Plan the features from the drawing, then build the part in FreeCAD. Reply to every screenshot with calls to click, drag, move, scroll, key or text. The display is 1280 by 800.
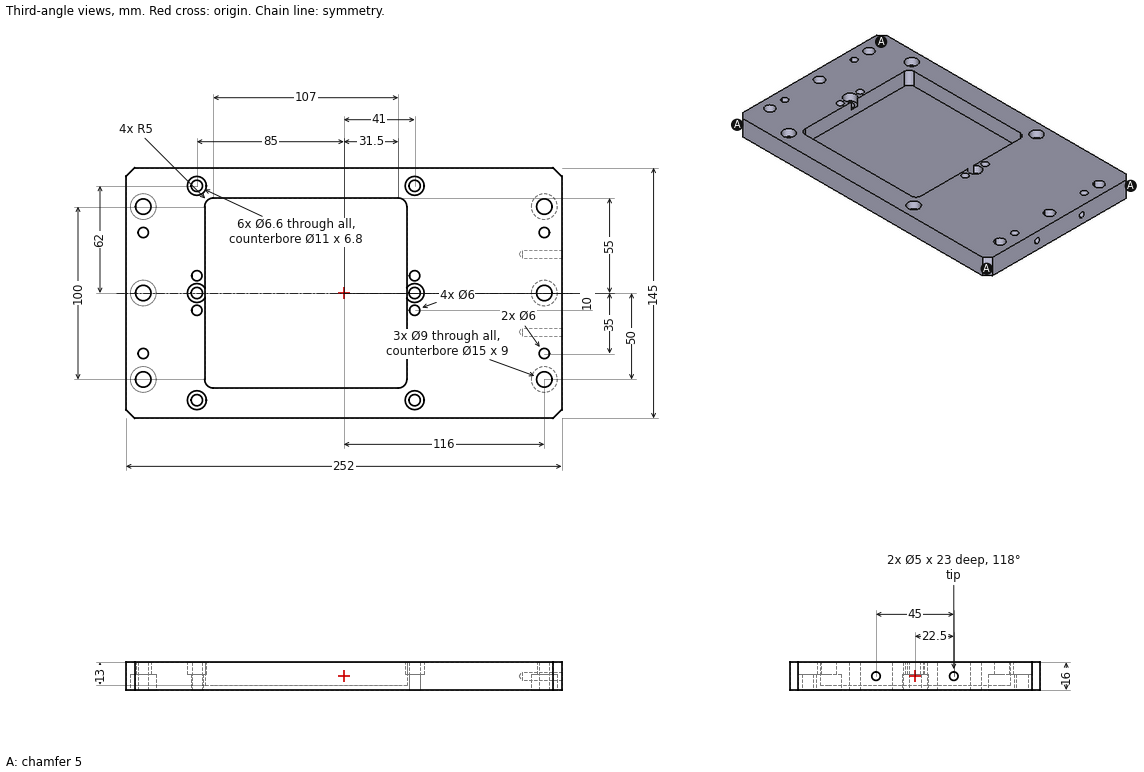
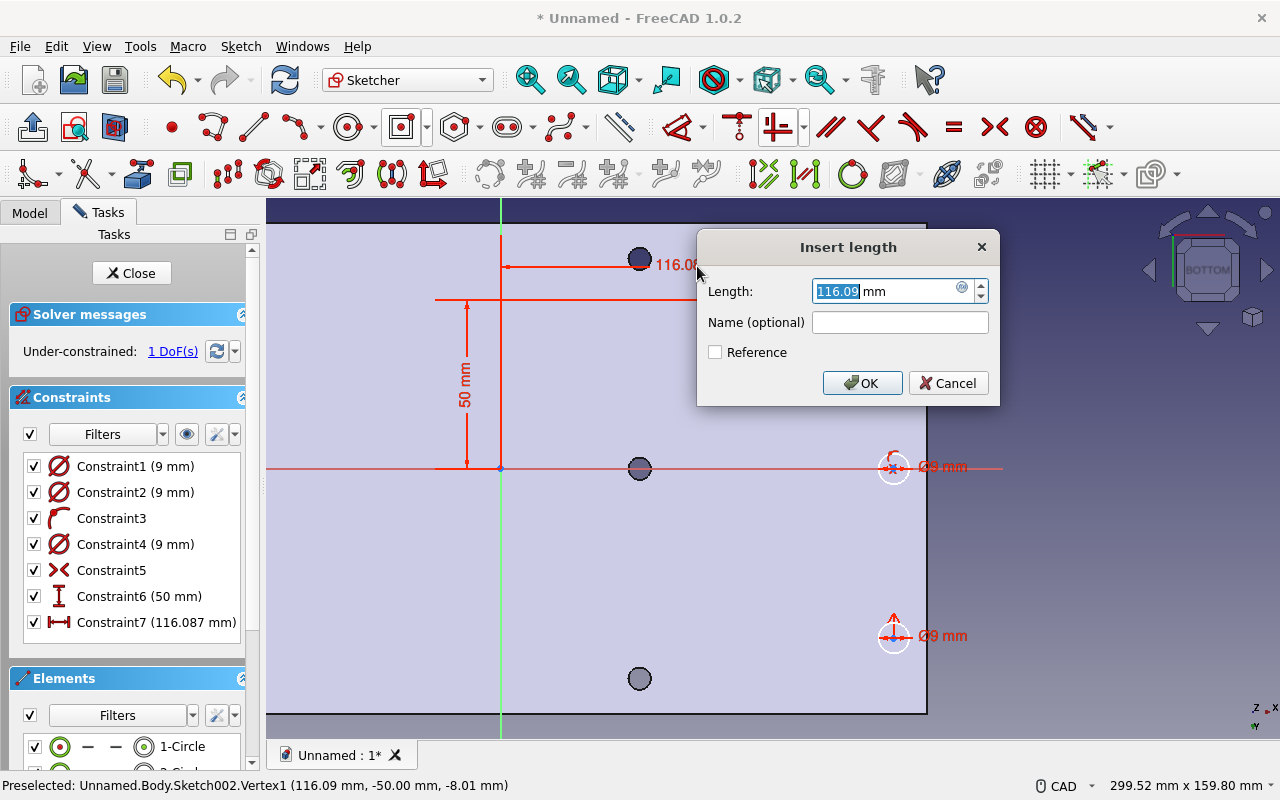
text(116)
key(Return)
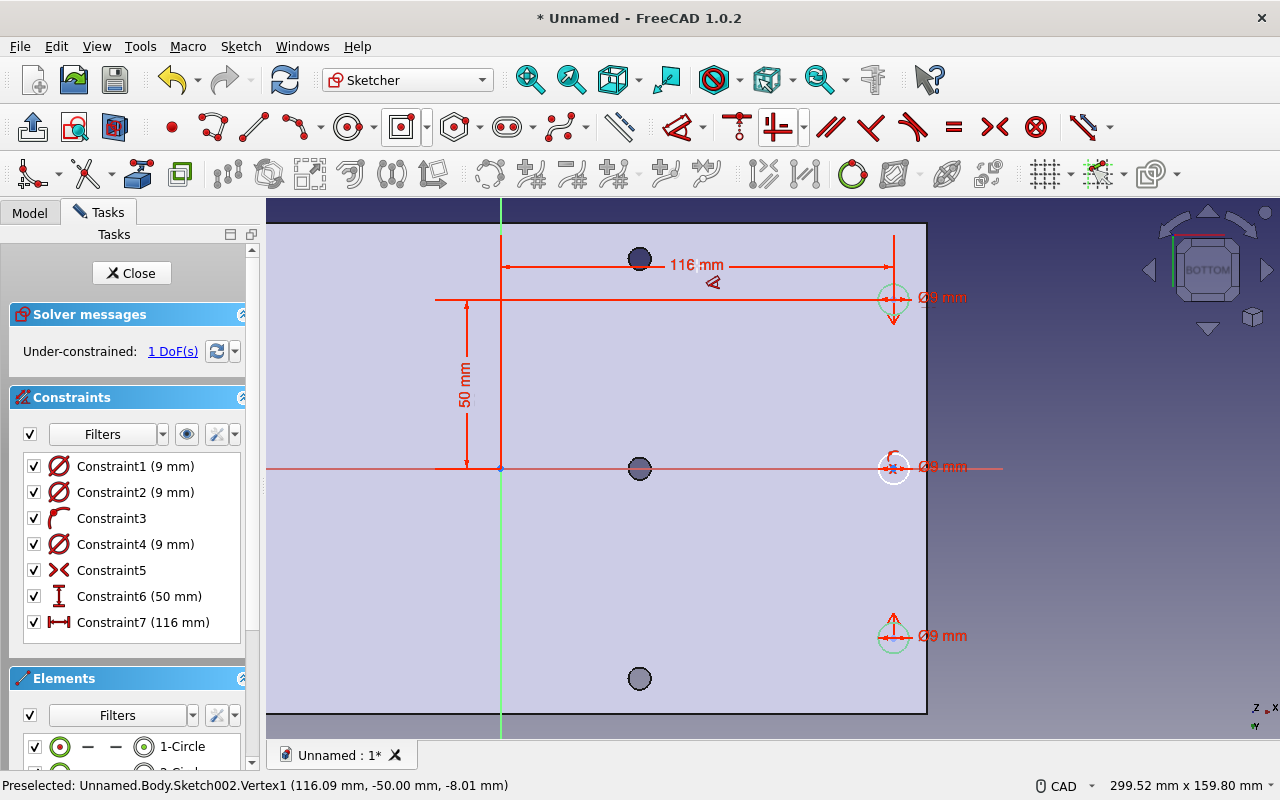
click(894, 469)
click(697, 503)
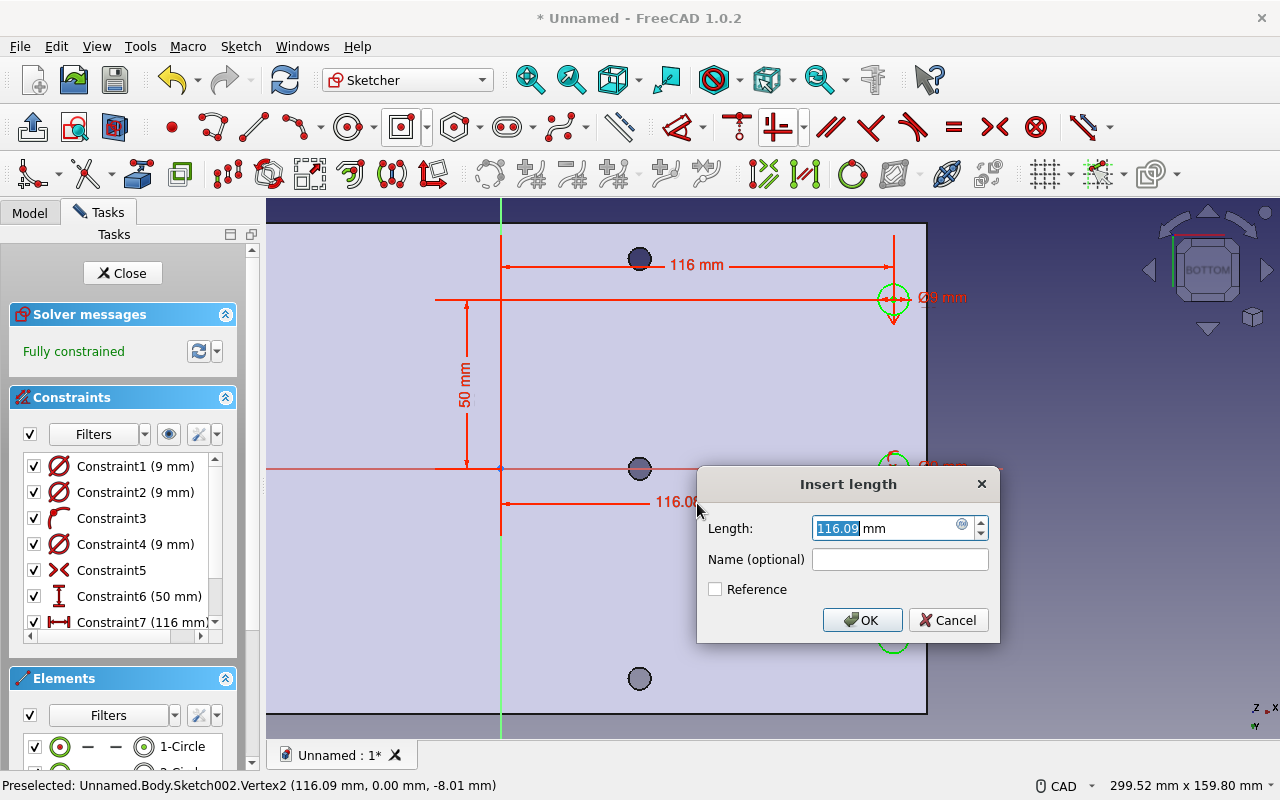
text(116)
key(Return)
key(Escape)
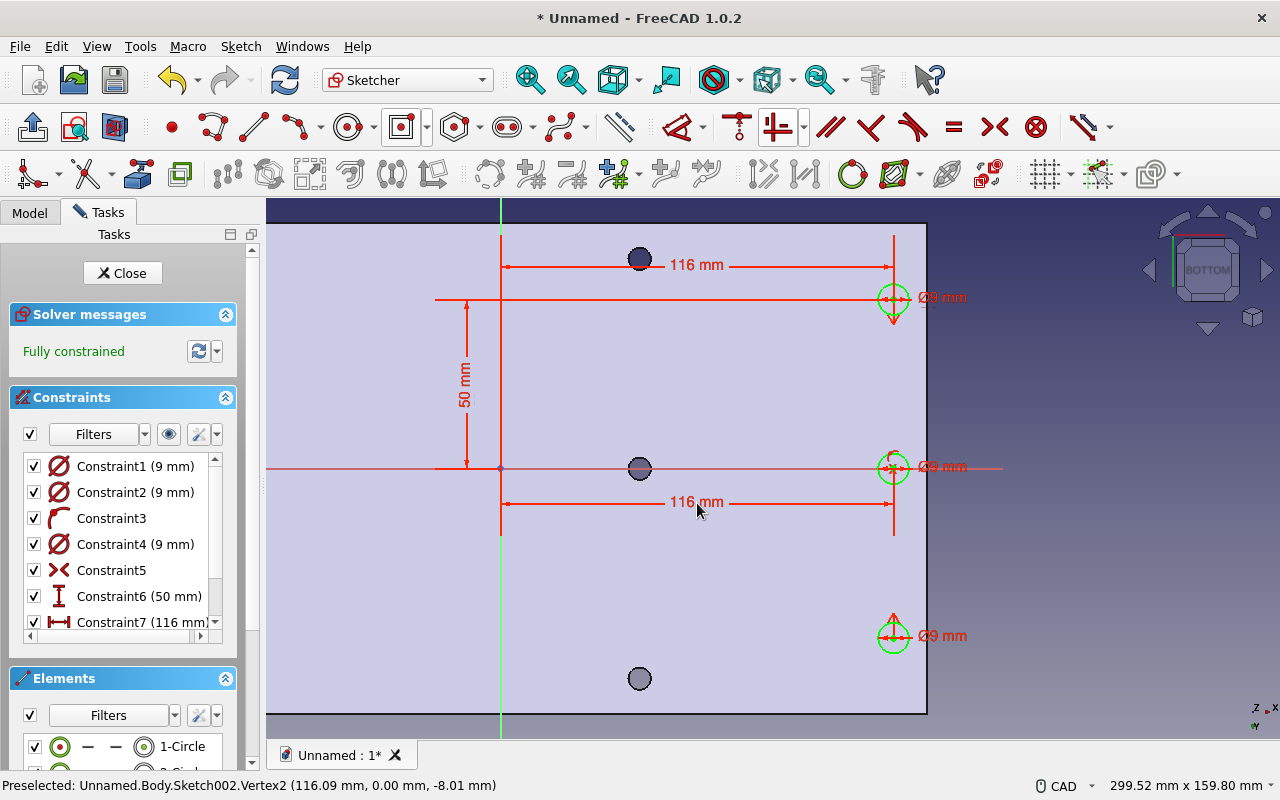
click(123, 273)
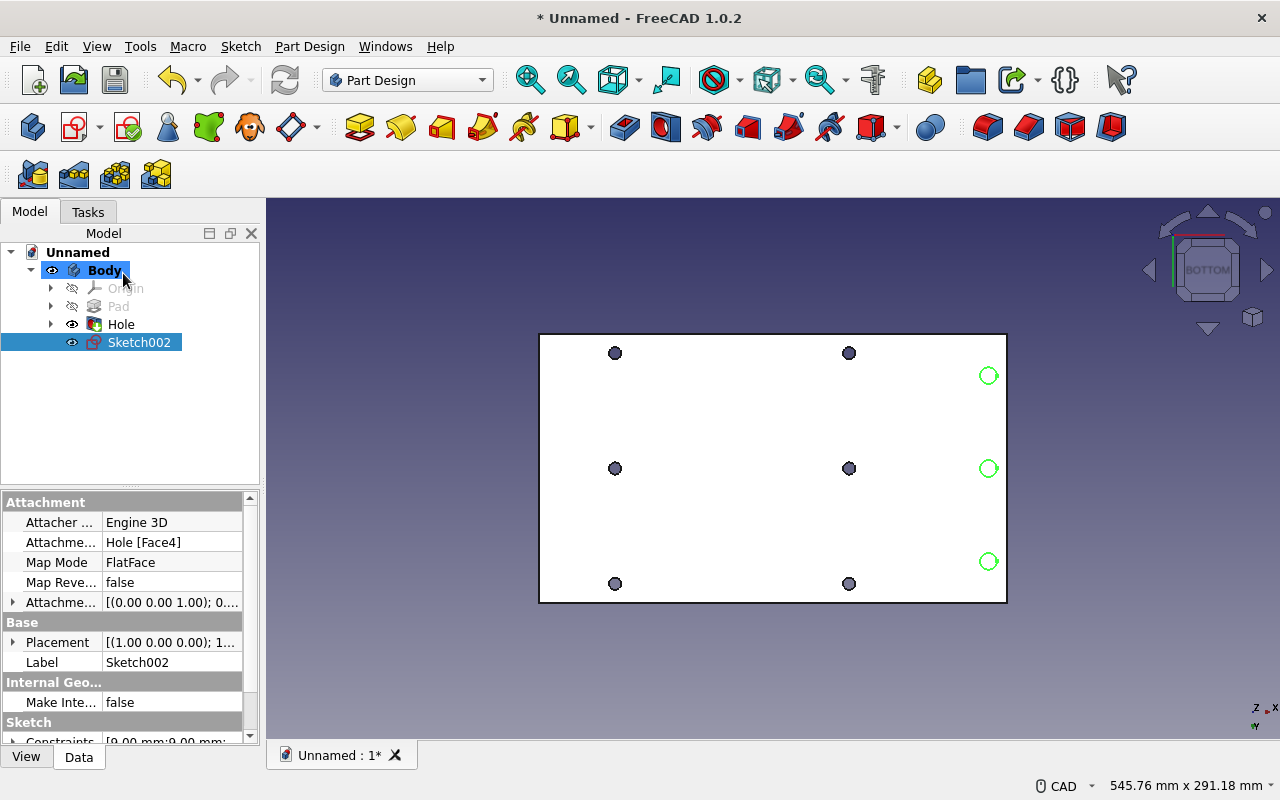
click(666, 128)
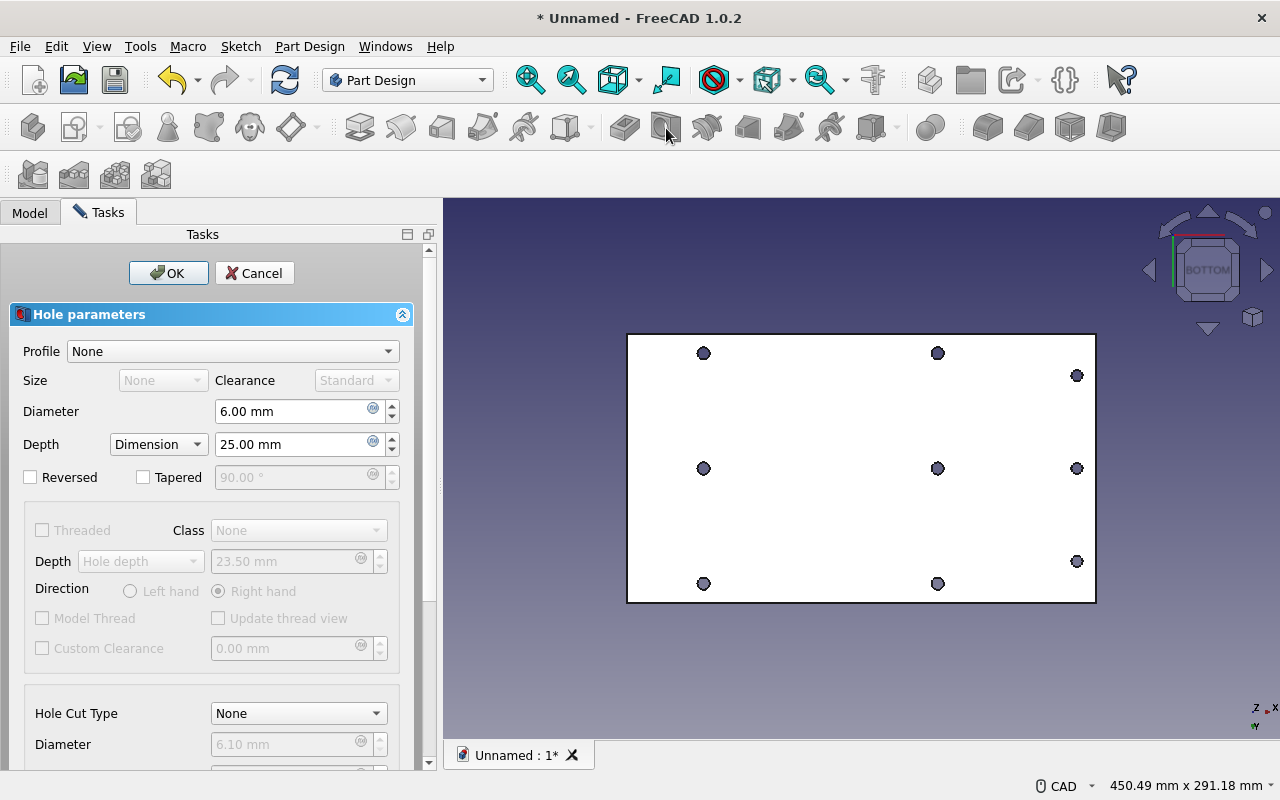
triple_click(300, 412)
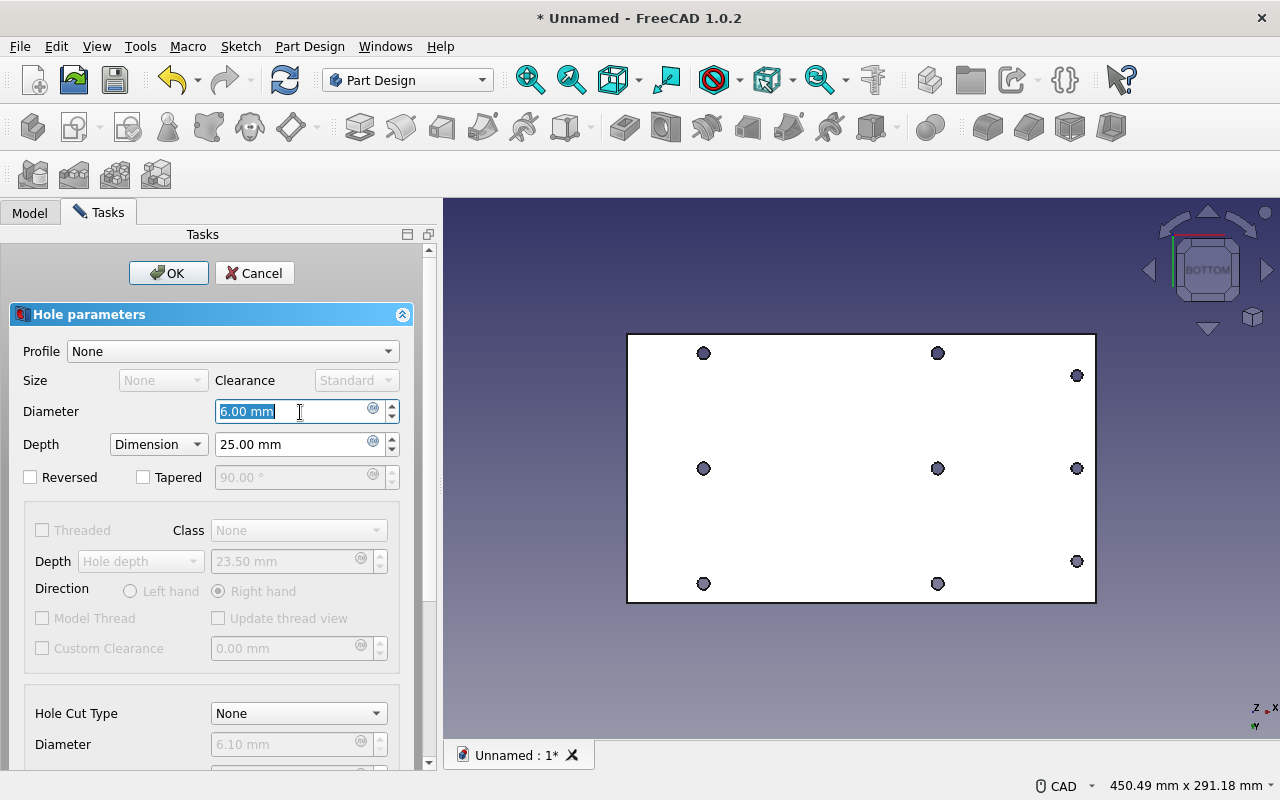
text(9)
key(Tab)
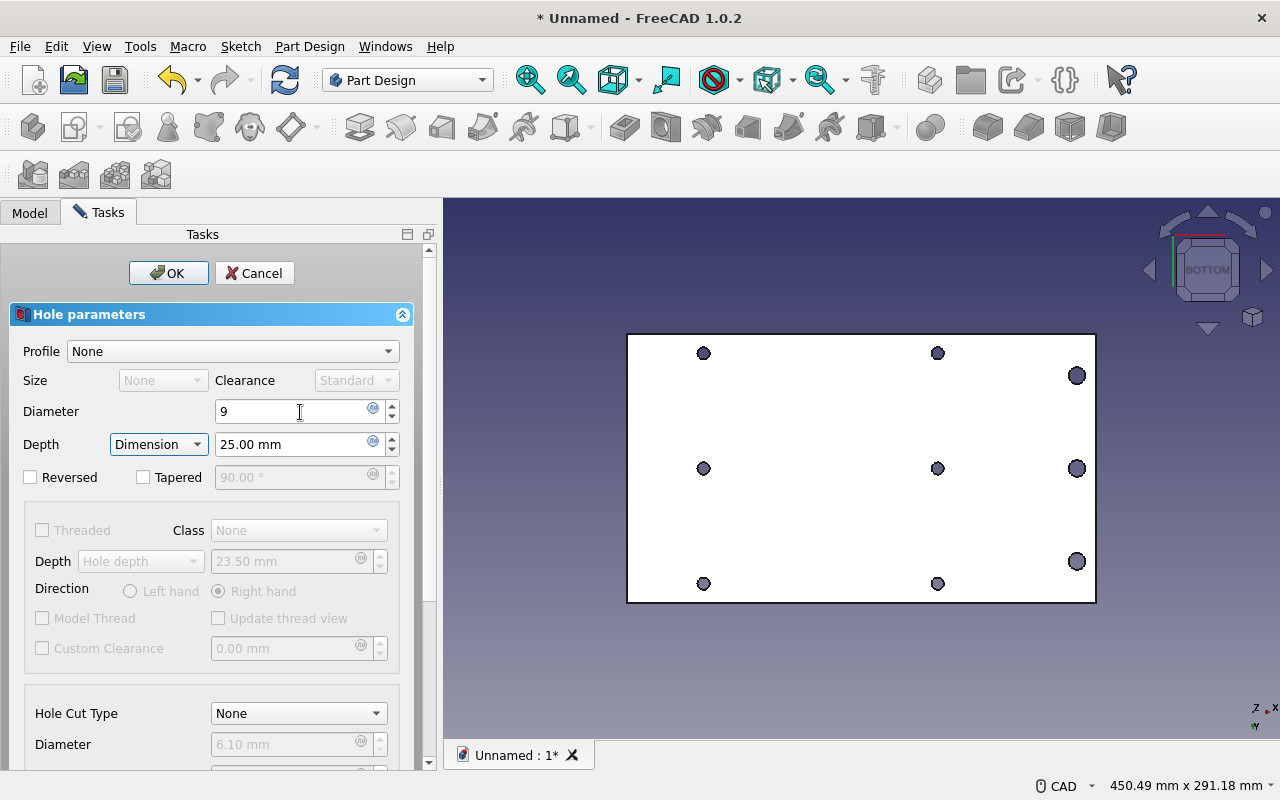
click(160, 444)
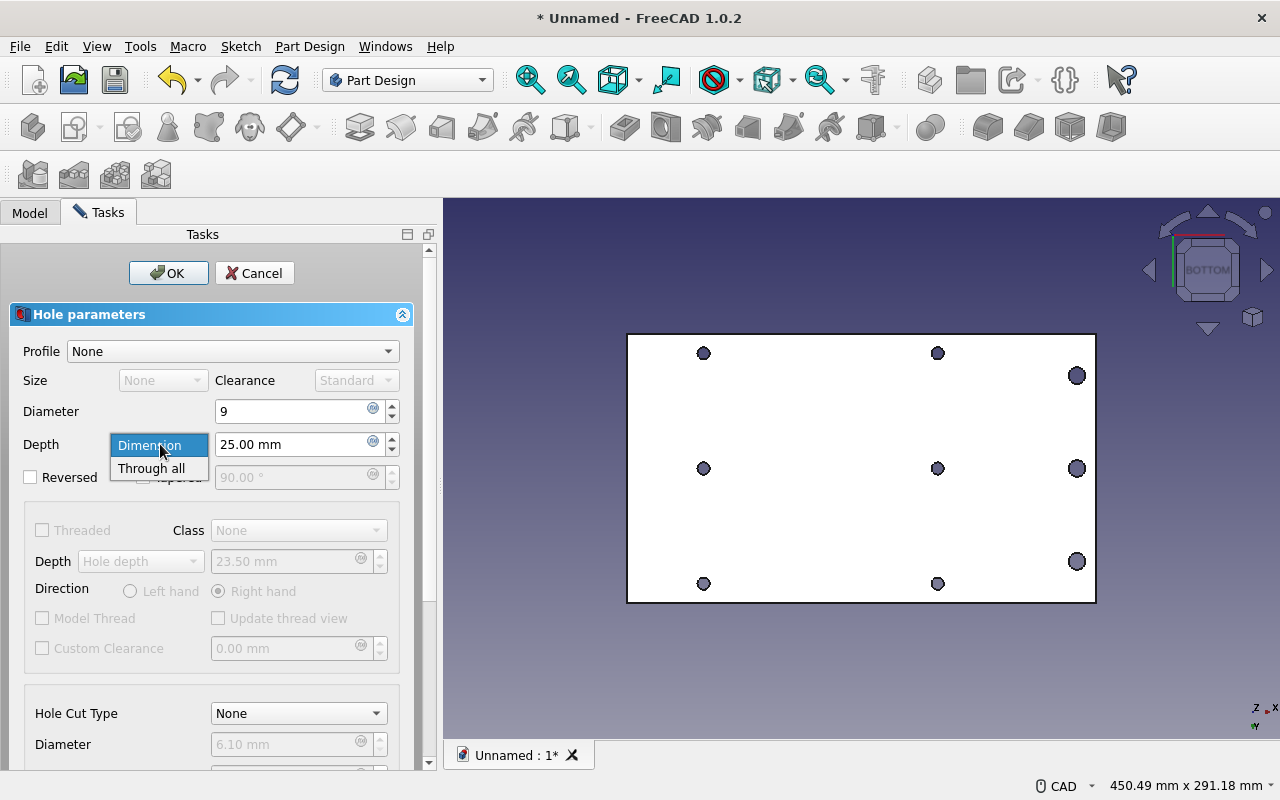
click(158, 468)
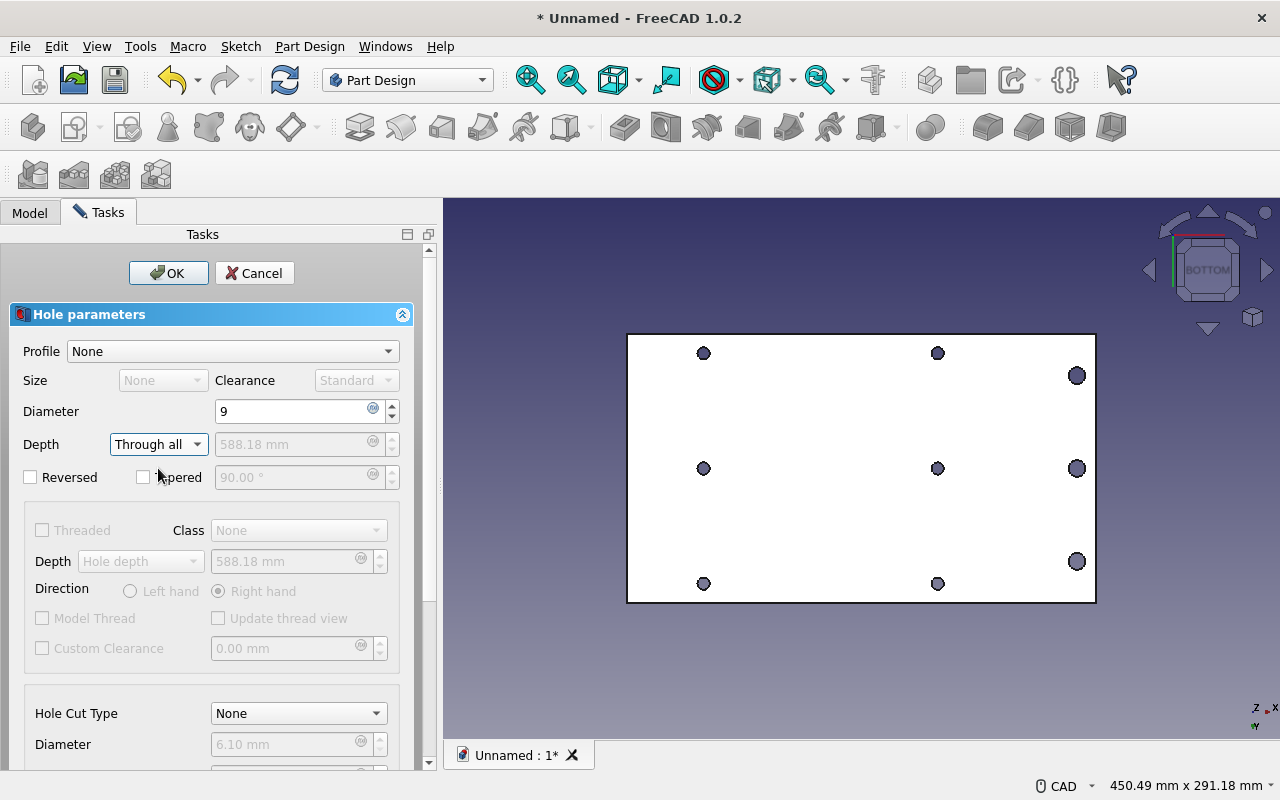
click(300, 714)